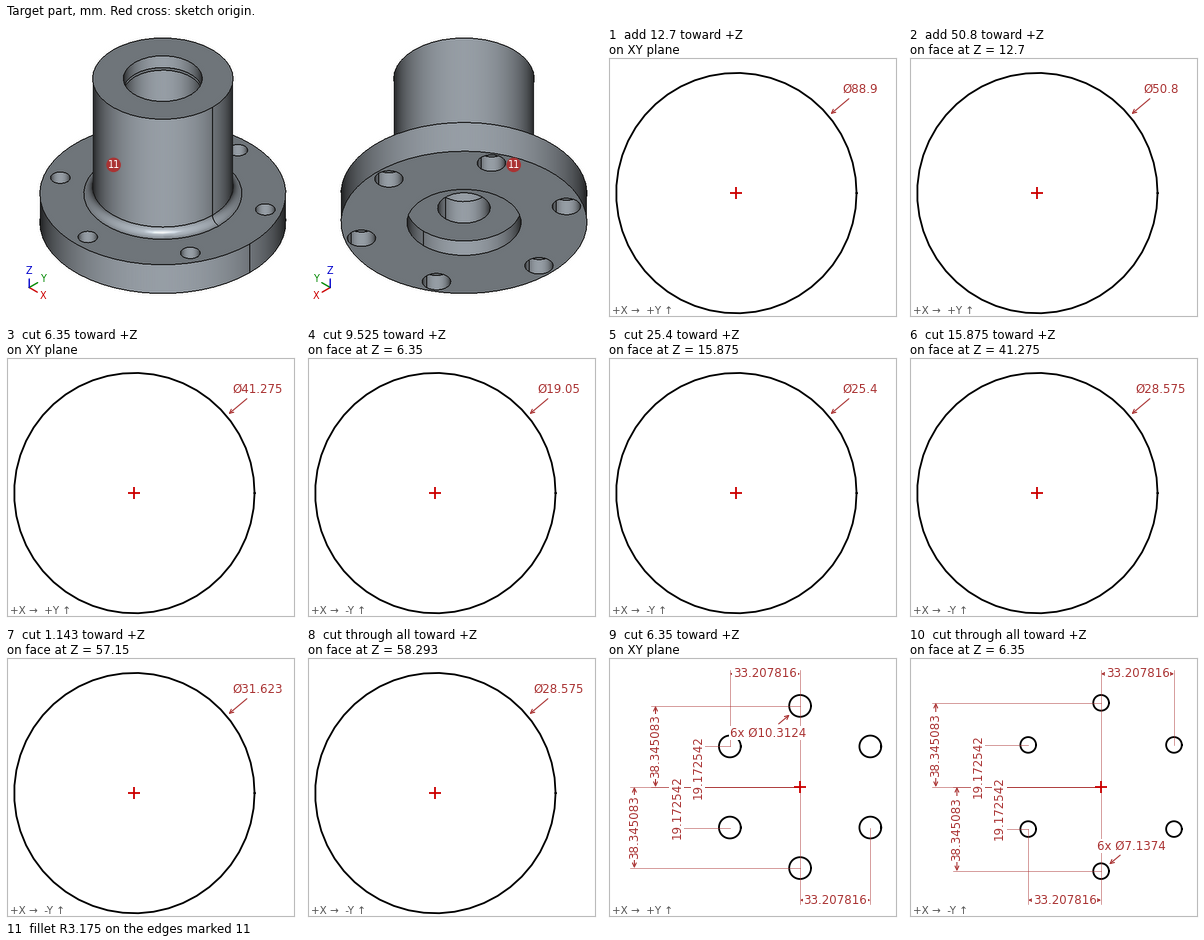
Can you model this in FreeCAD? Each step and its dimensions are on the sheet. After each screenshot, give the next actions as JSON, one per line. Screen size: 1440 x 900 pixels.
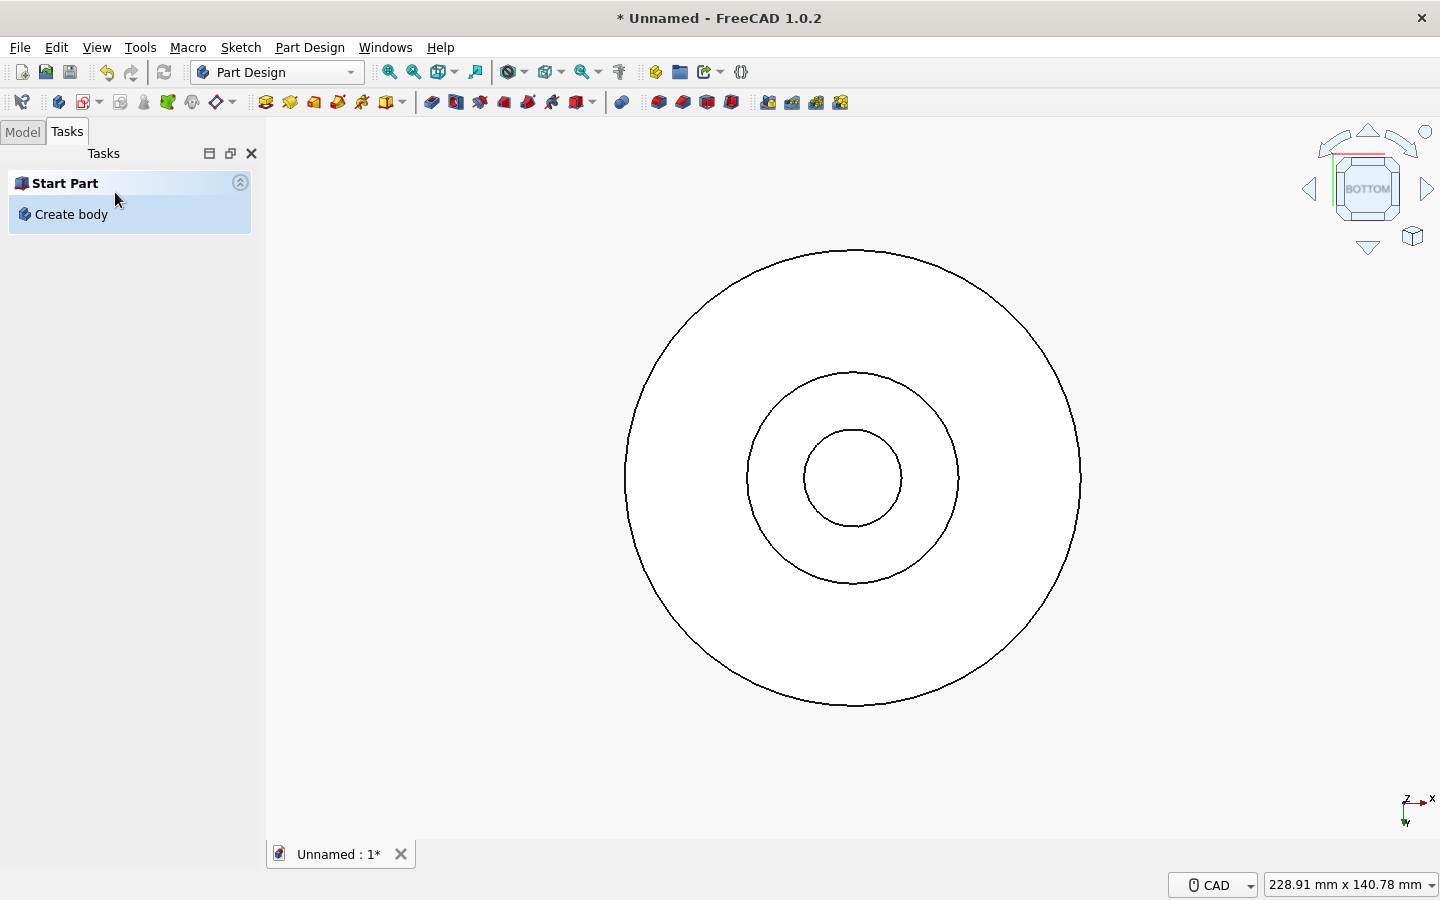
{"action": "left_click", "coordinate": [853, 477]}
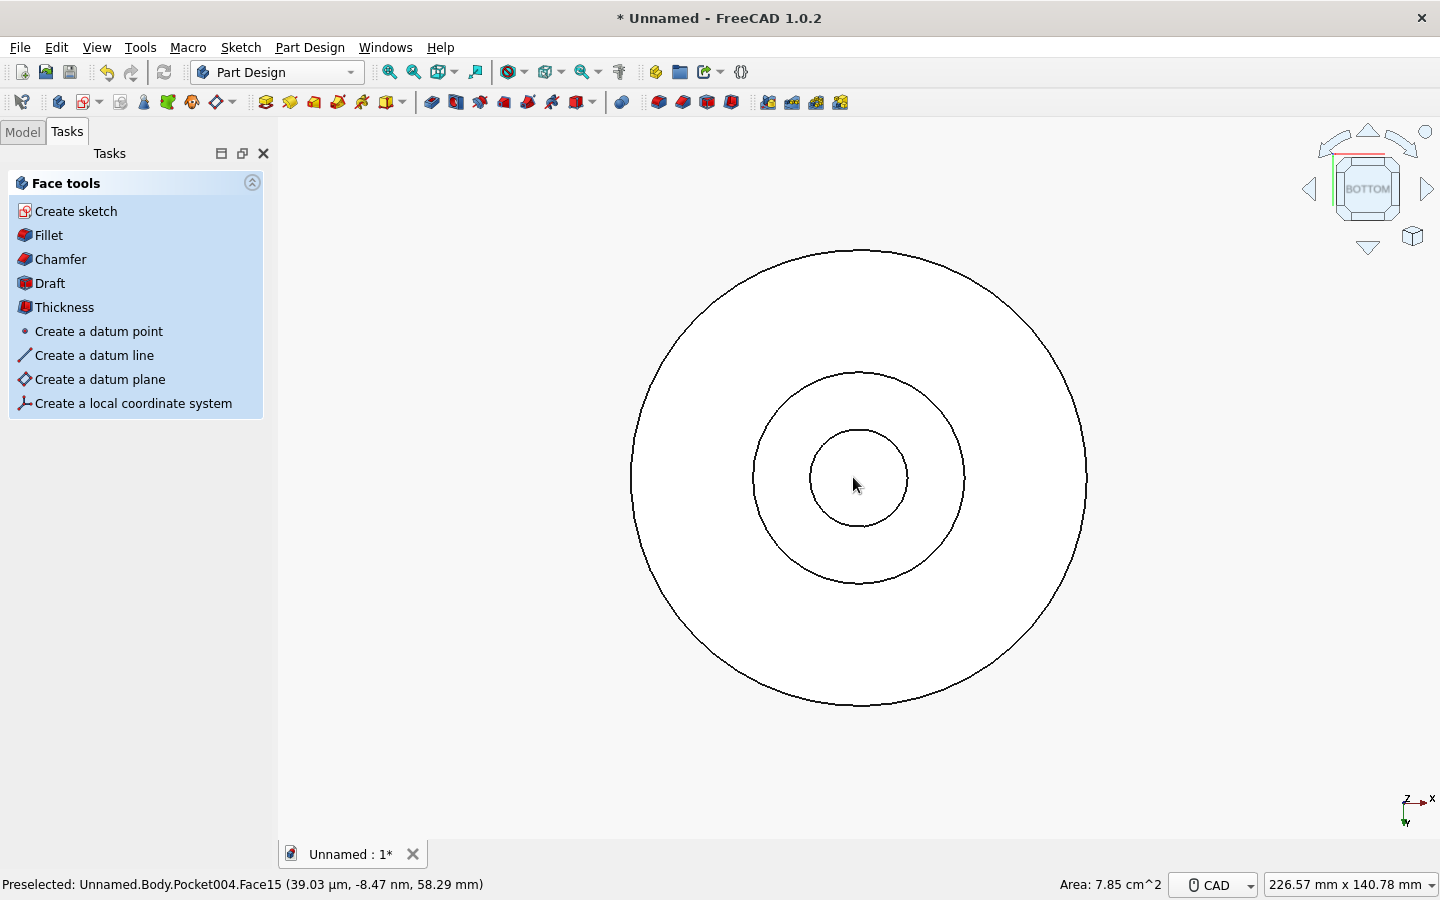
{"action": "left_click", "coordinate": [84, 102]}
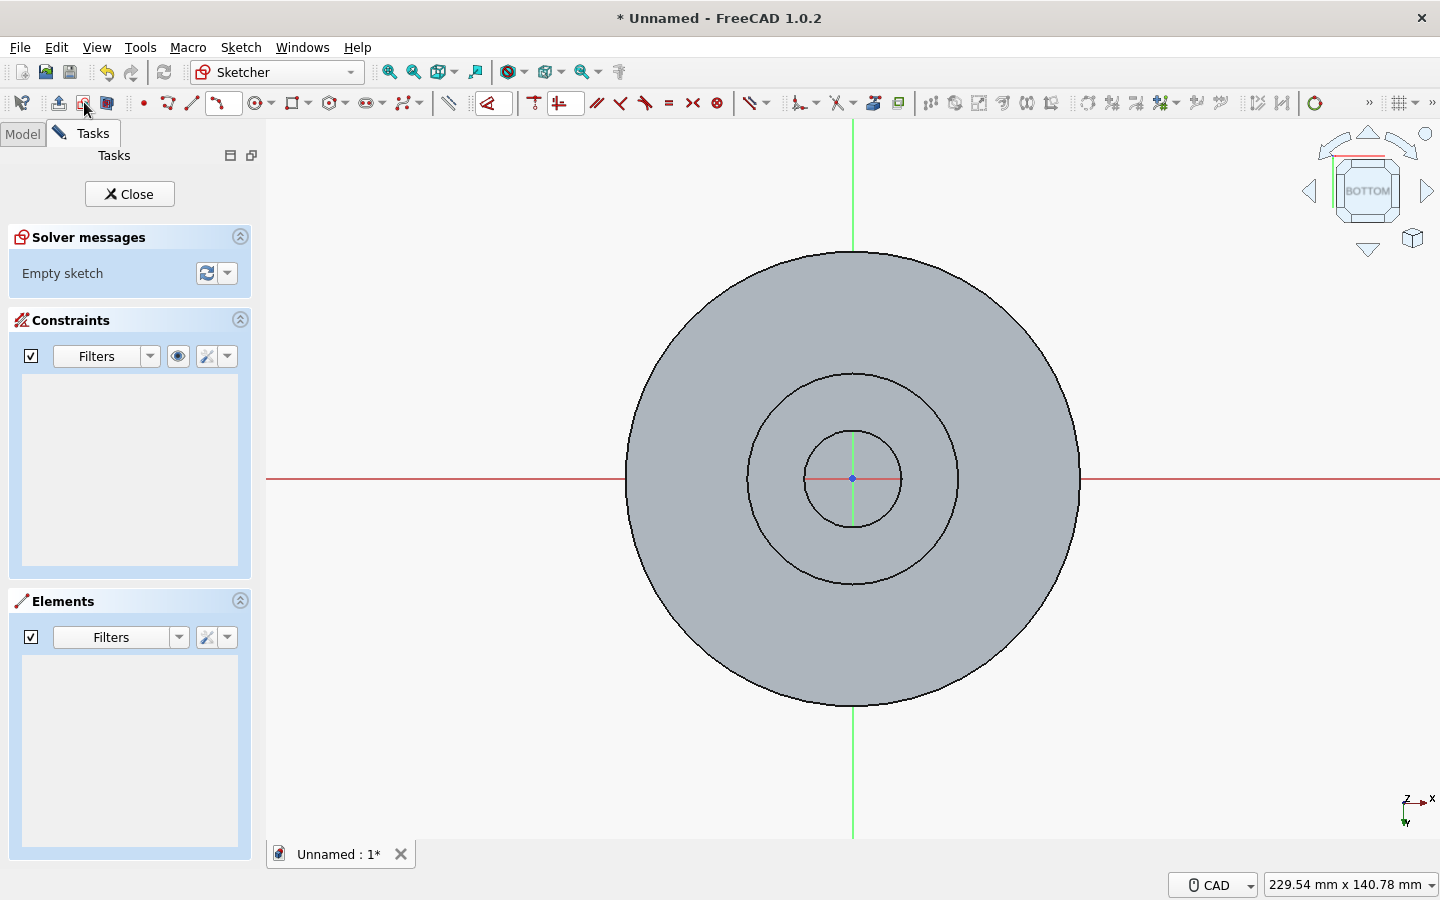
{"action": "left_click", "coordinate": [108, 104]}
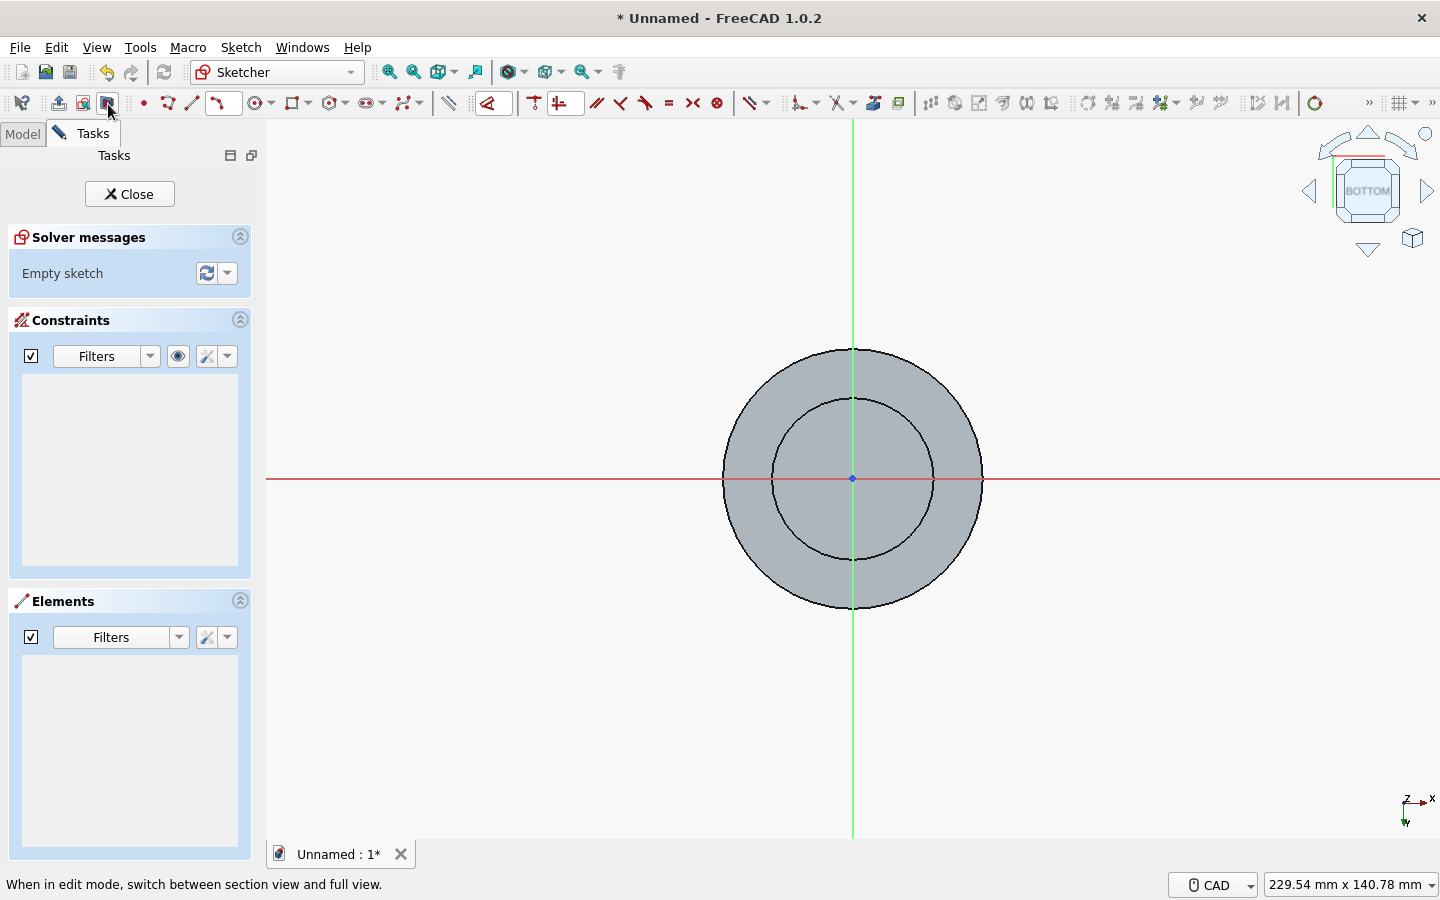
{"action": "scroll", "coordinate": [882, 479], "scroll_direction": "up", "scroll_amount": 6}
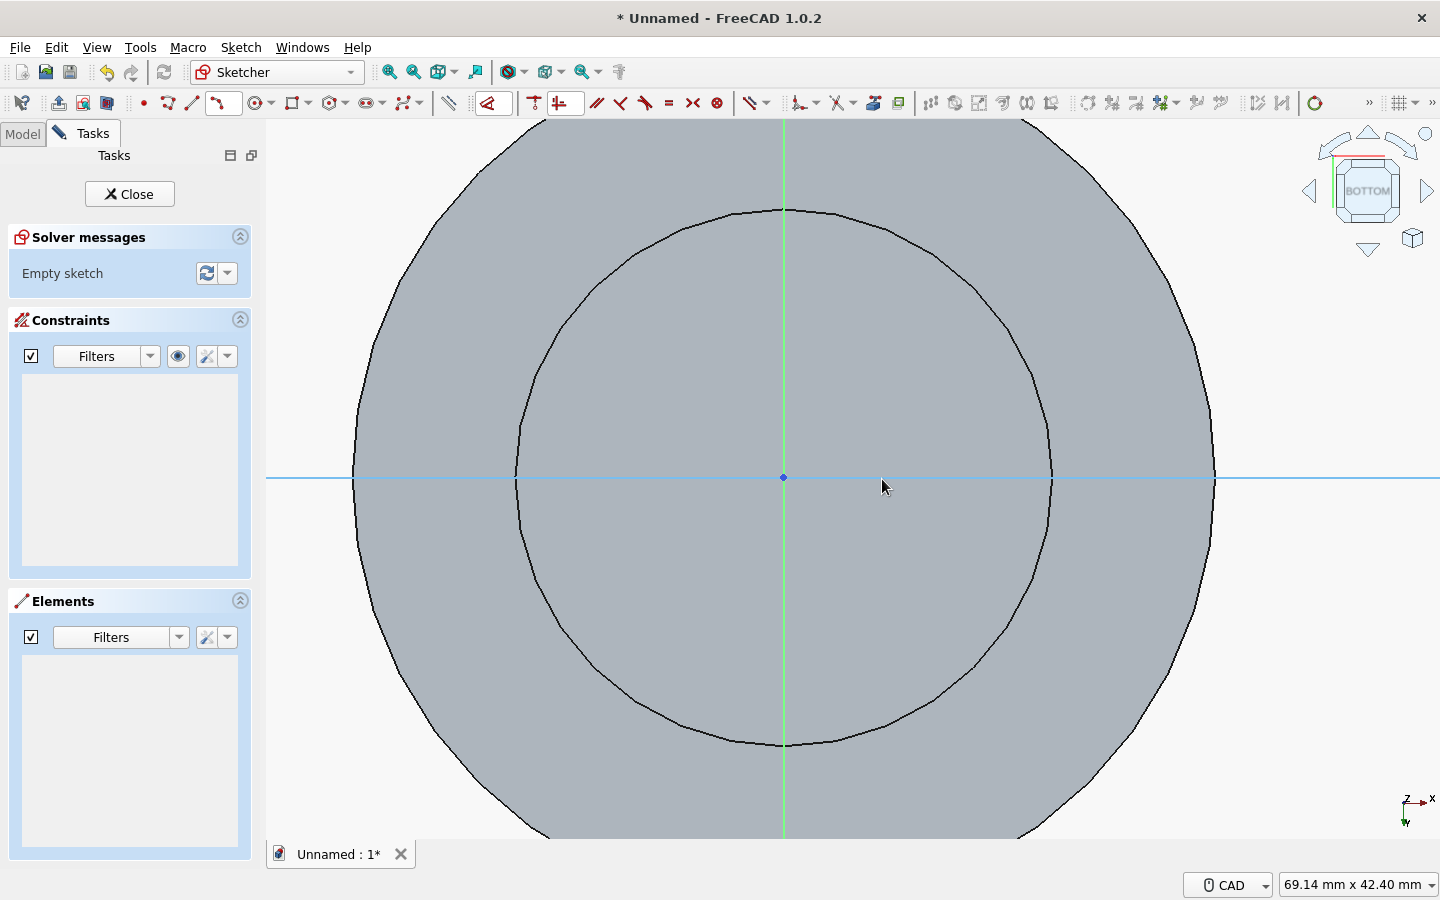
{"action": "key", "text": "g c"}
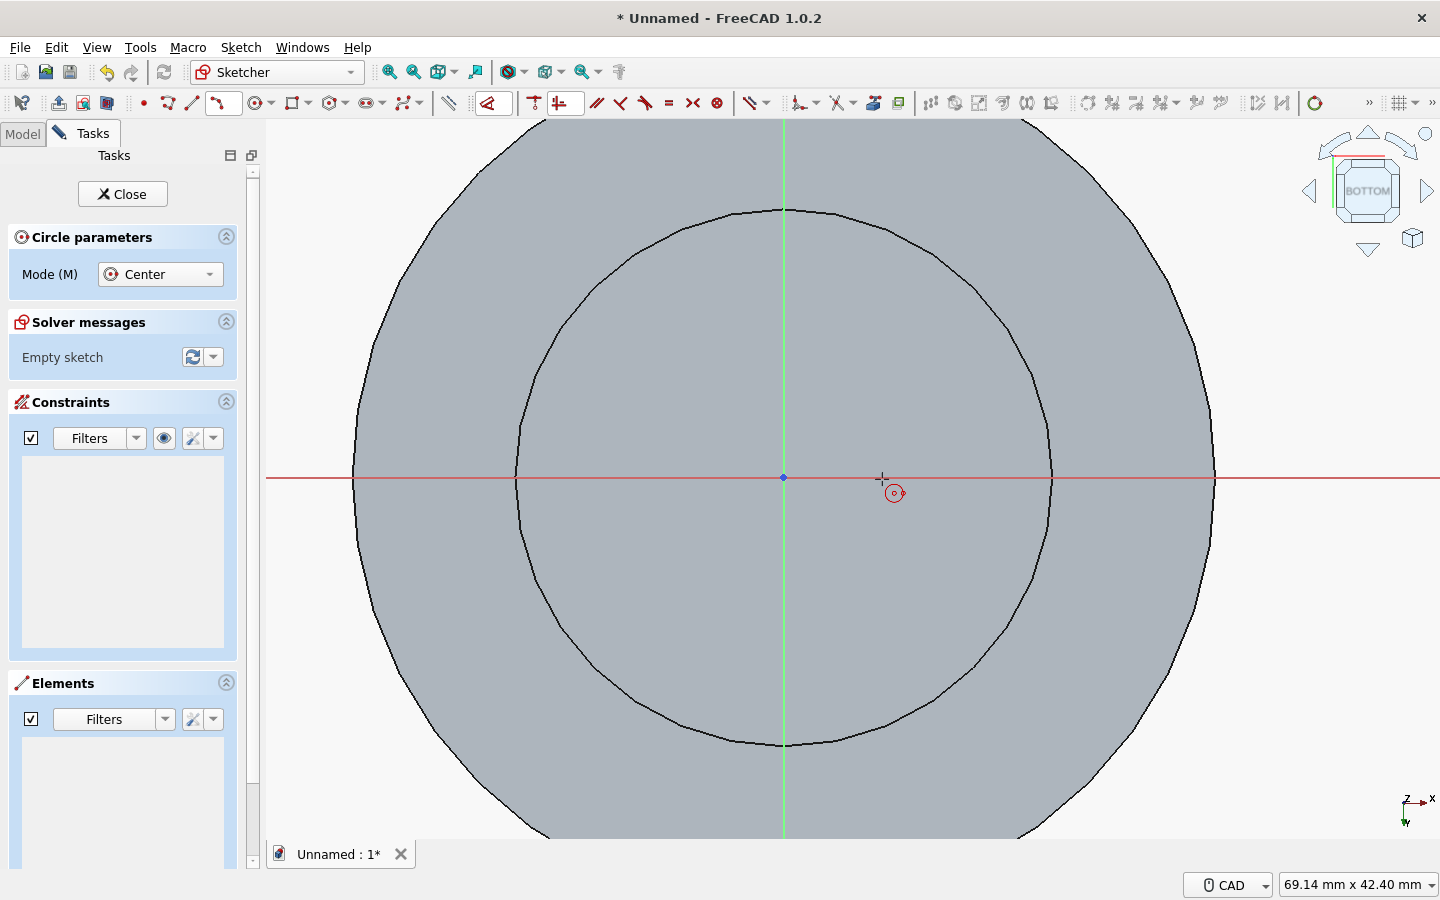
{"action": "left_click", "coordinate": [784, 478]}
{"action": "mouse_move", "coordinate": [955, 306]}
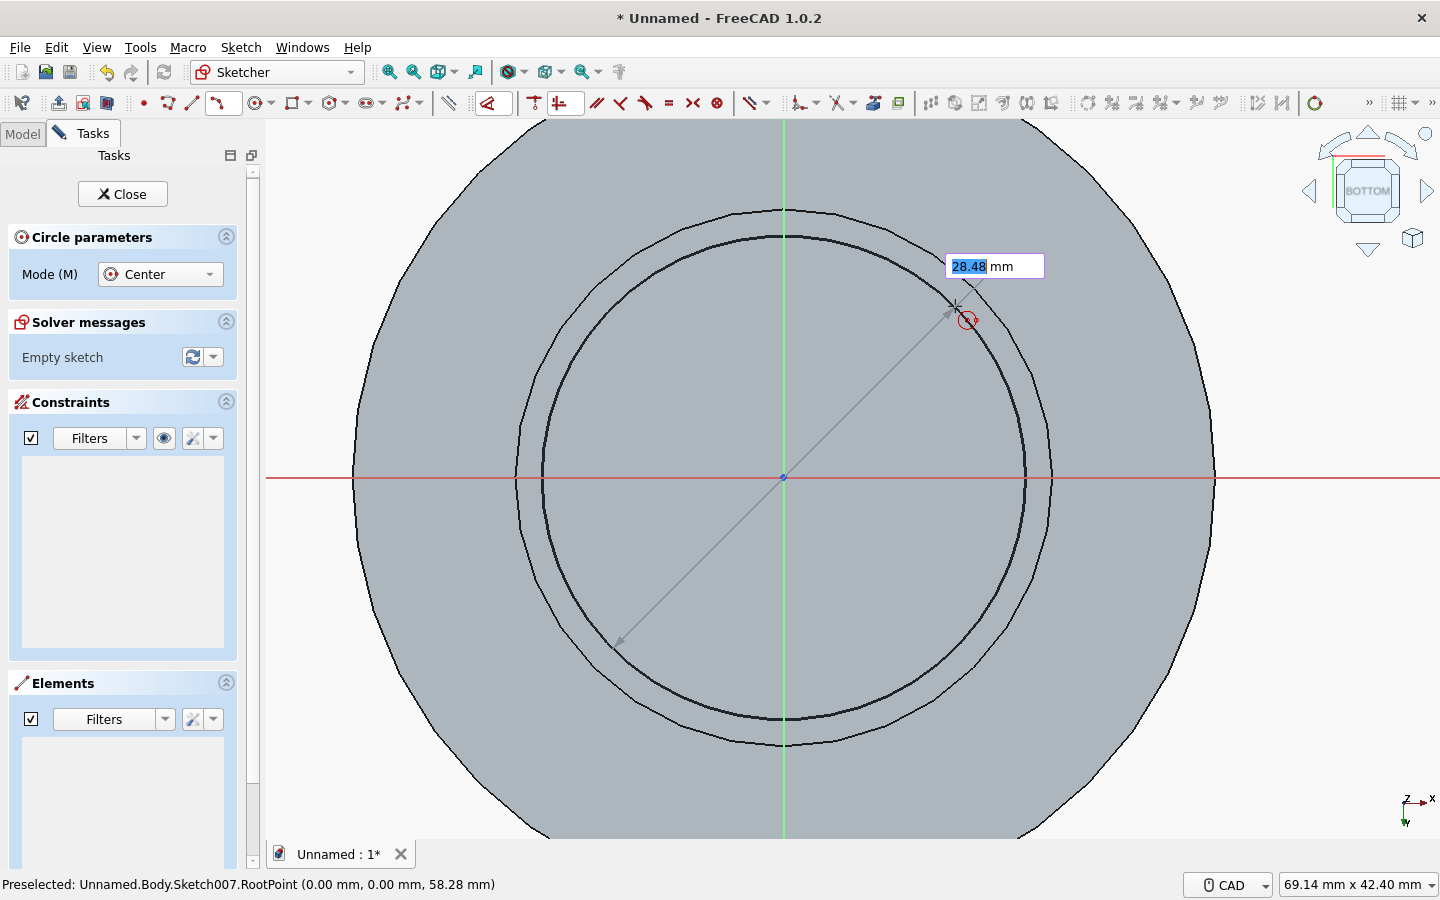
{"action": "type", "text": "28.575"}
{"action": "key", "text": "Return"}
{"action": "key", "text": "Escape"}